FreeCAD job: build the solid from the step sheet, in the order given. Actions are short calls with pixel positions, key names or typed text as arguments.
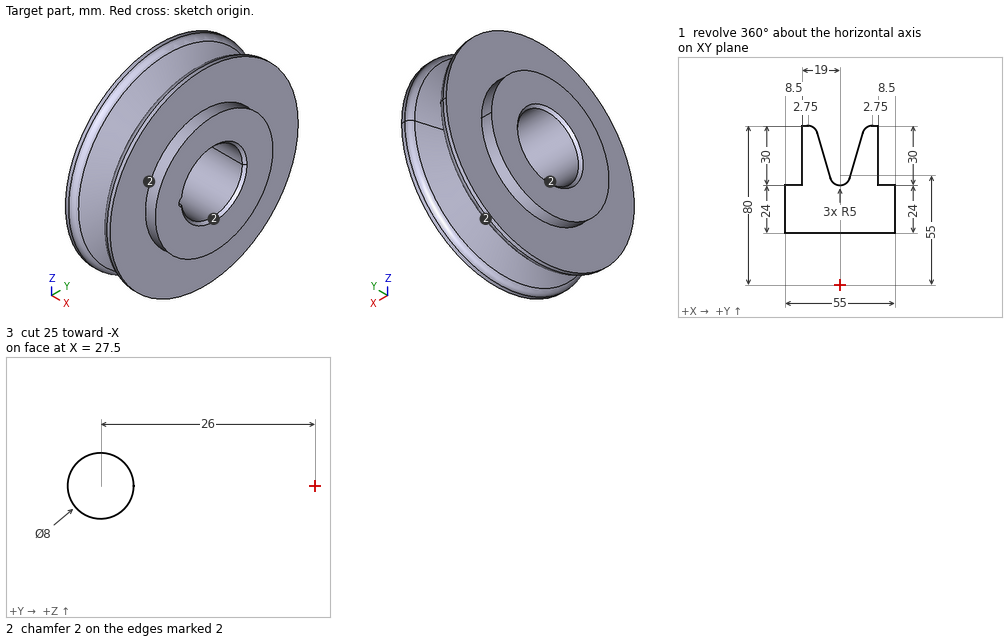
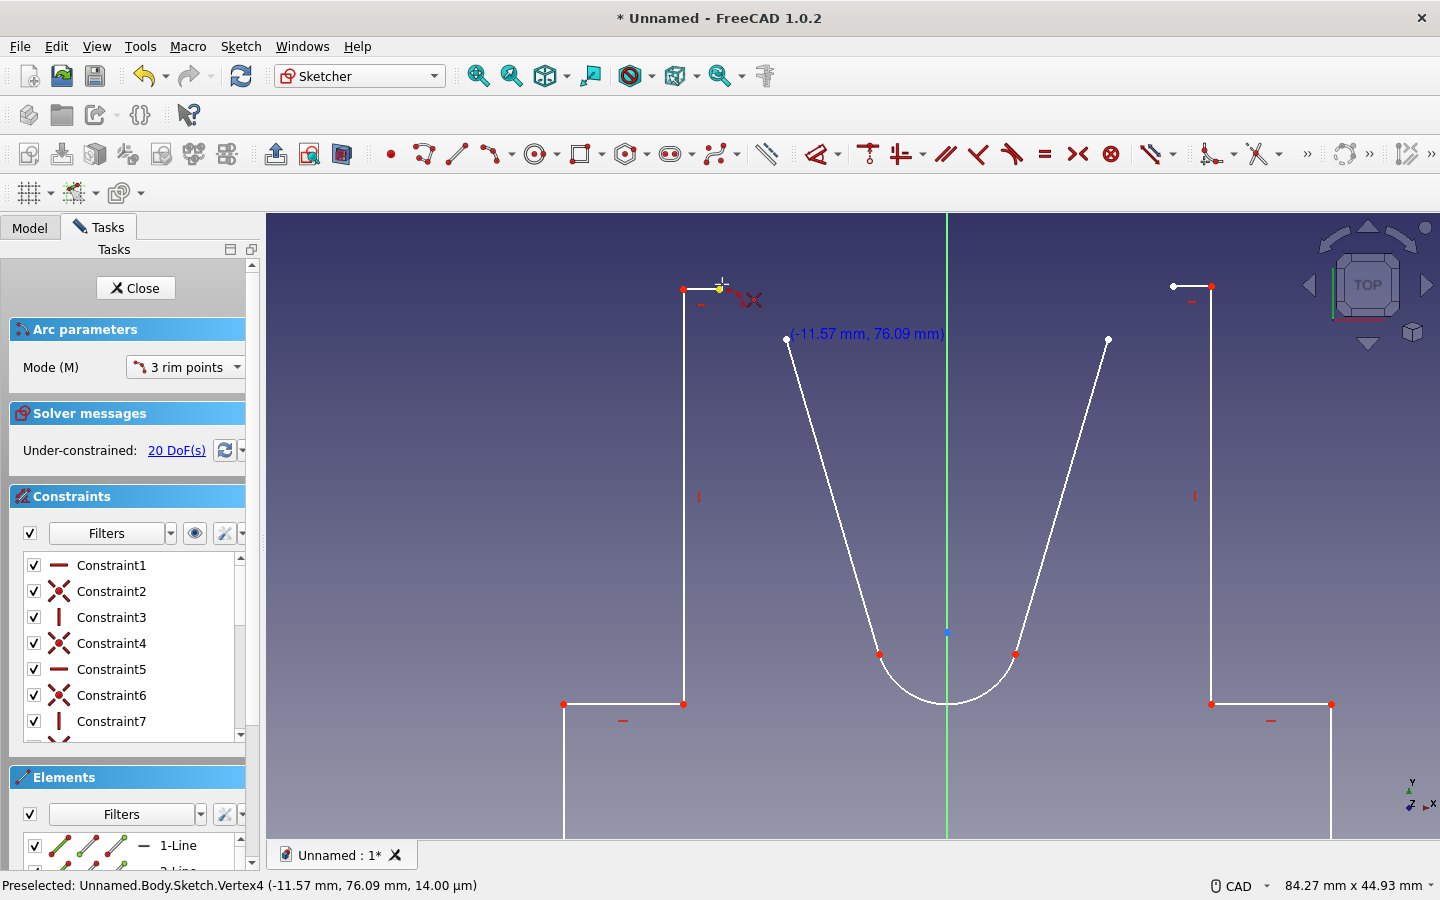
click(720, 289)
click(763, 298)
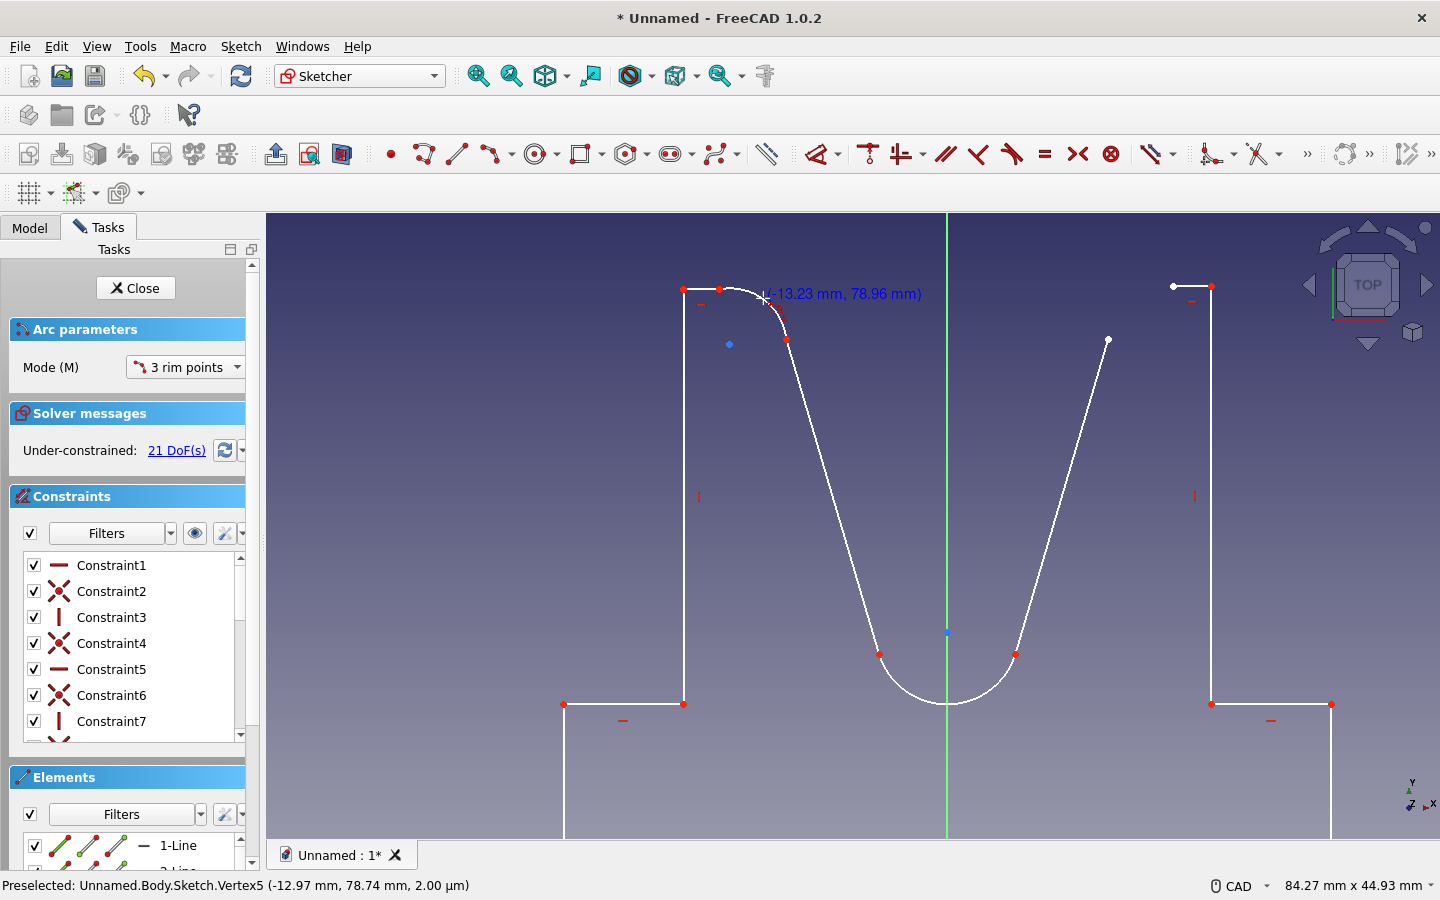
click(1173, 286)
click(1108, 339)
click(1132, 298)
key(Escape)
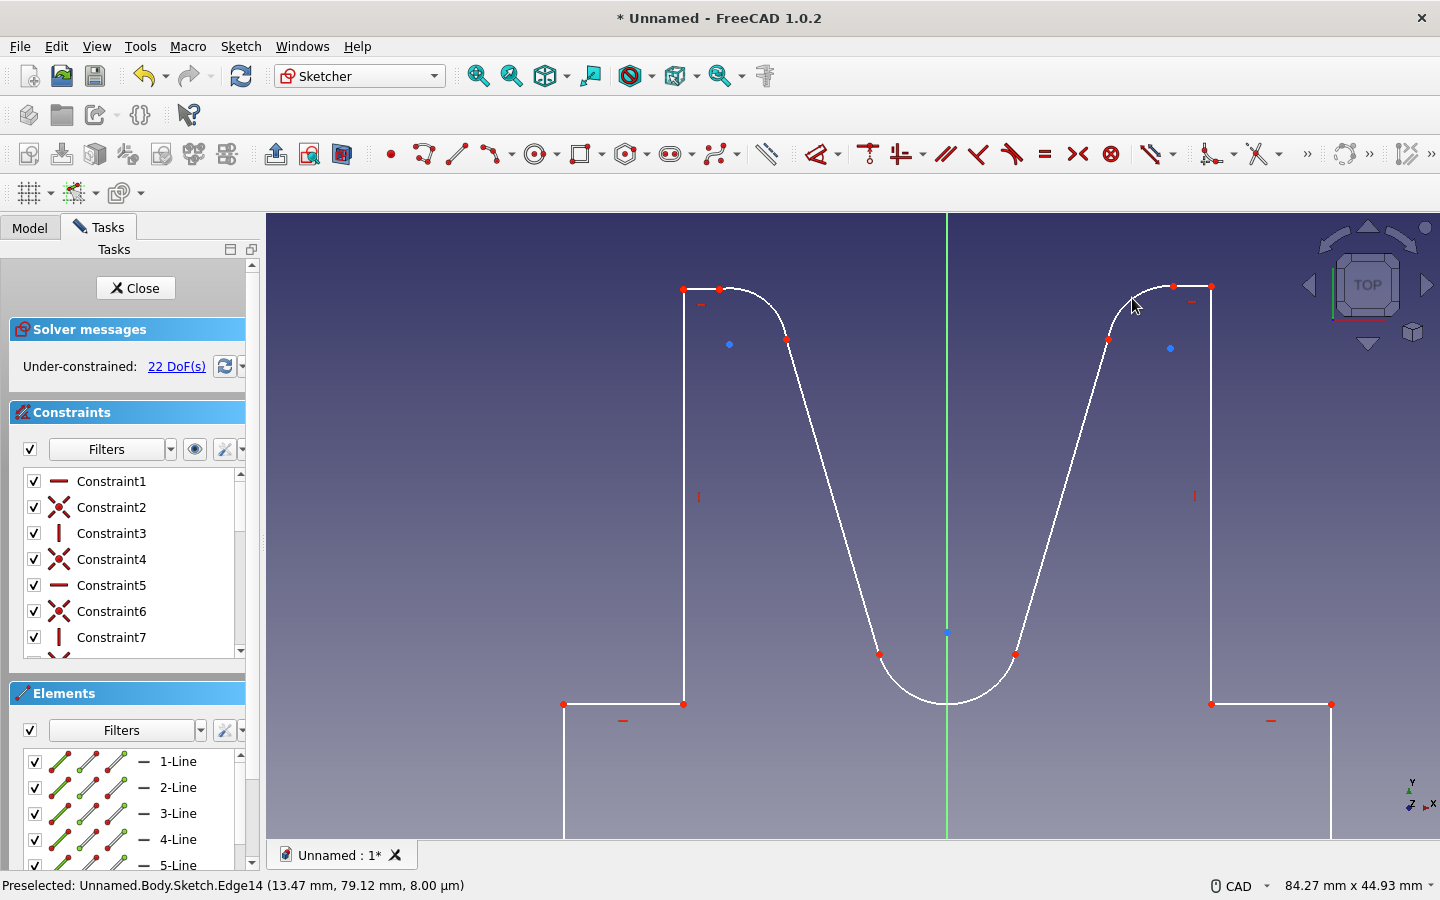
click(1080, 434)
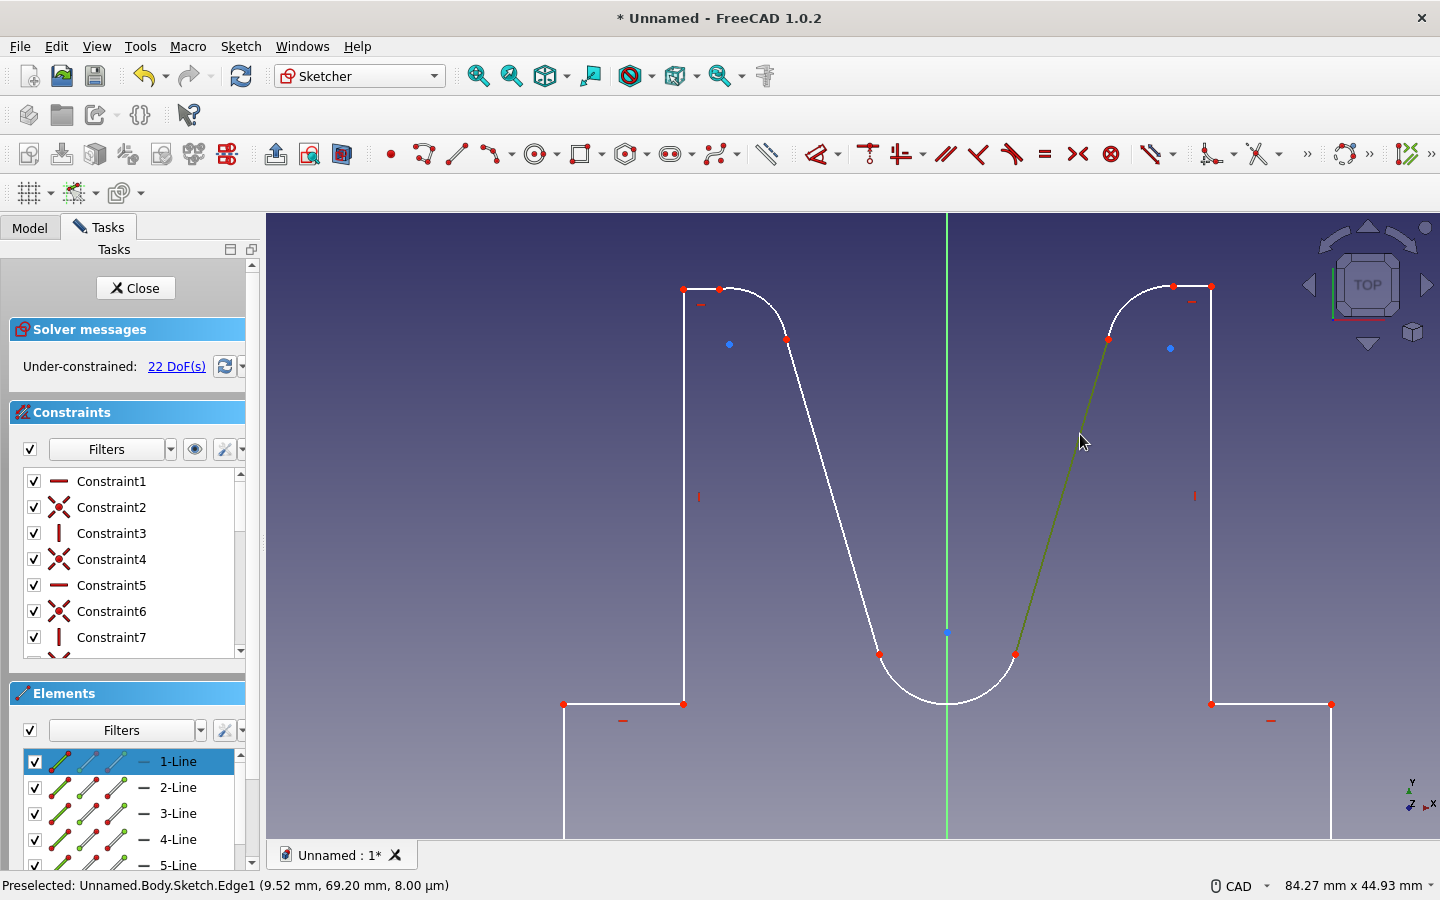
click(913, 695)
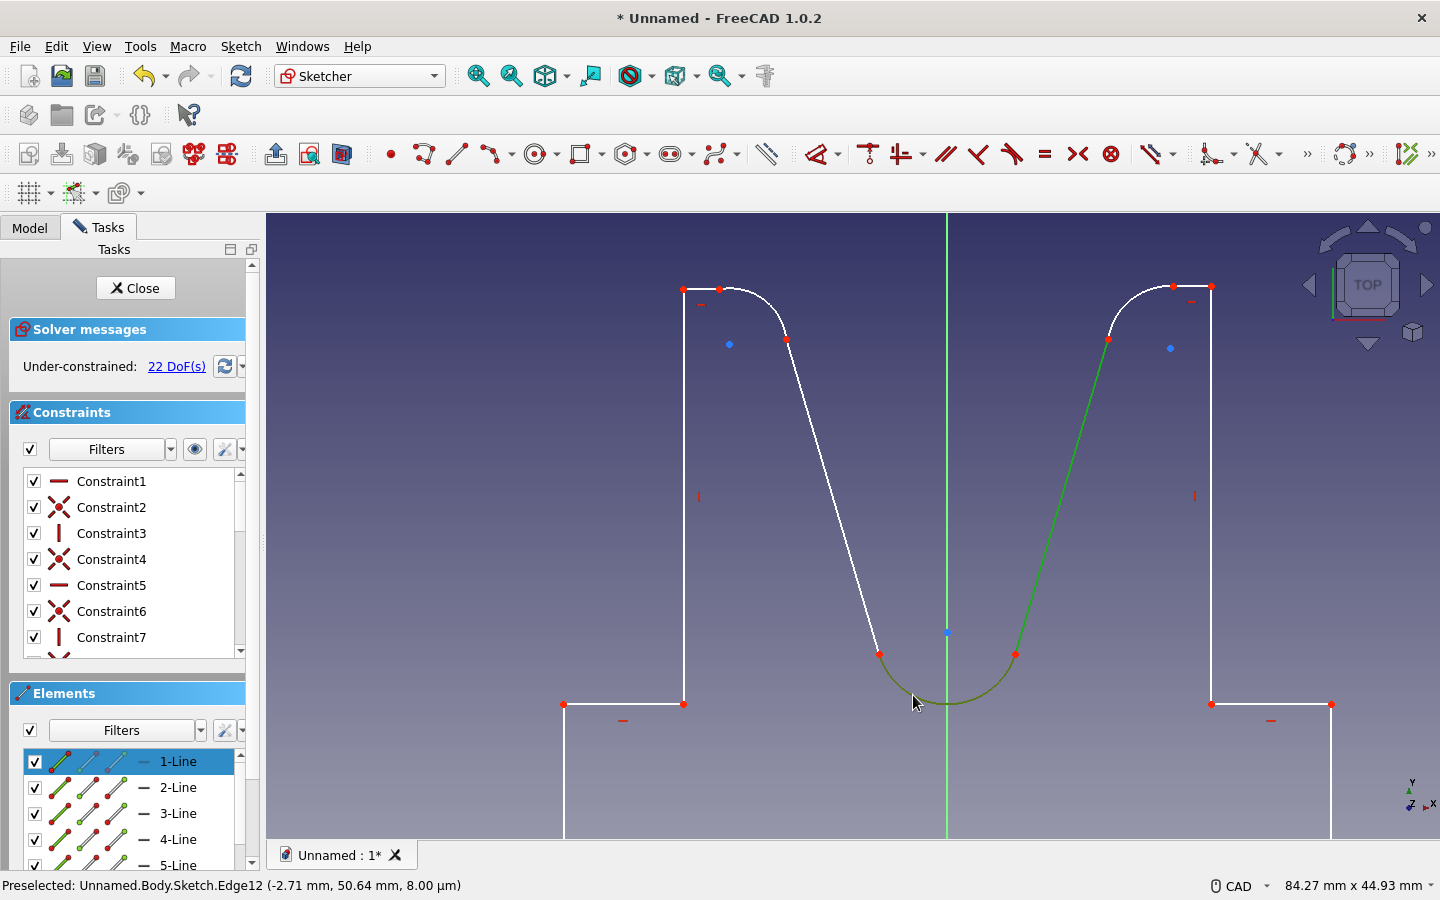
key(t)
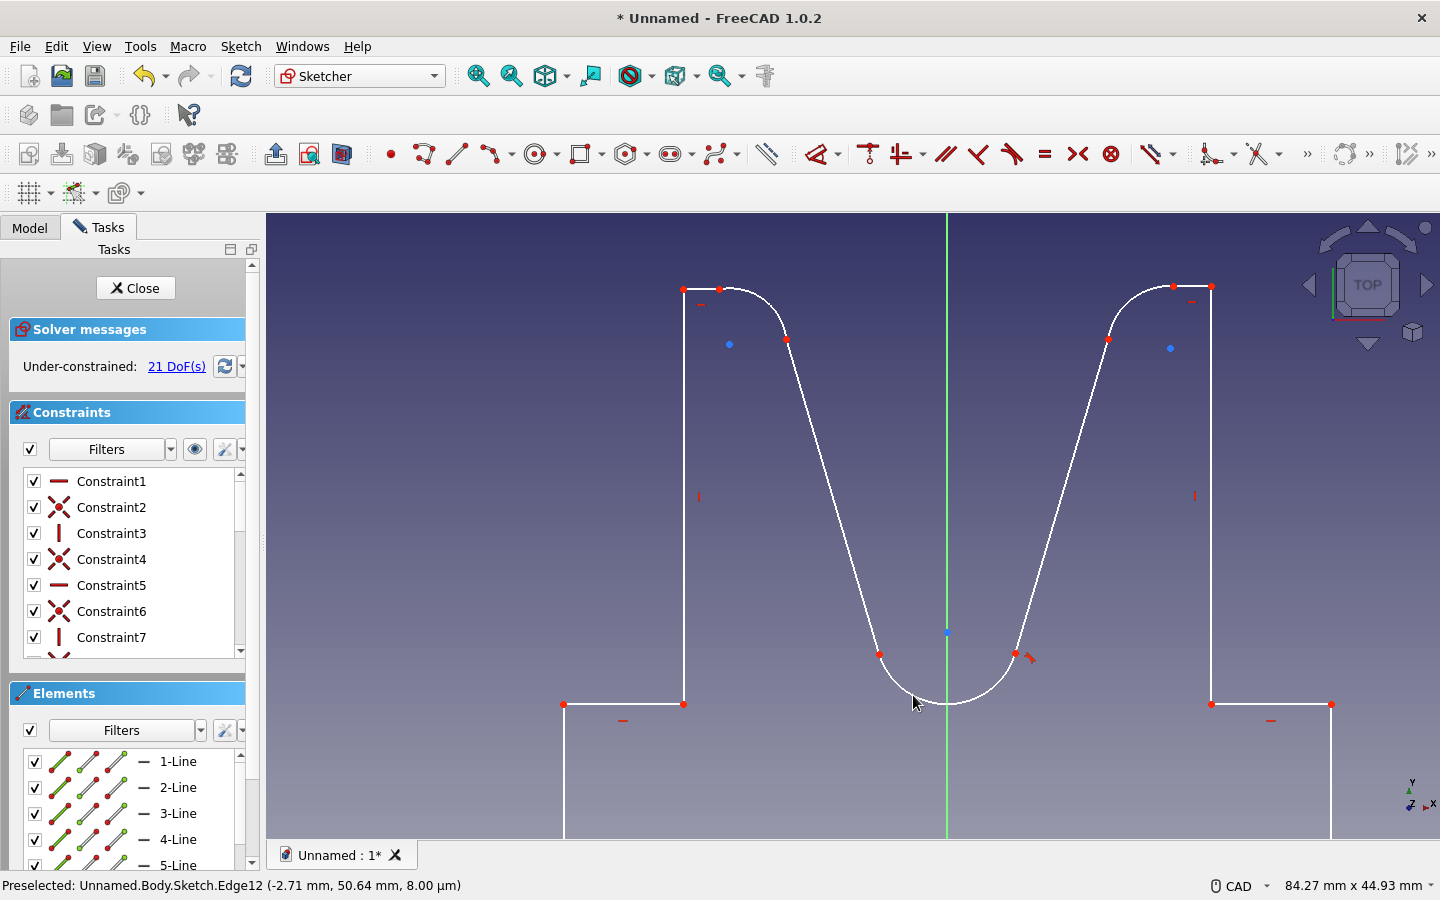
click(1080, 433)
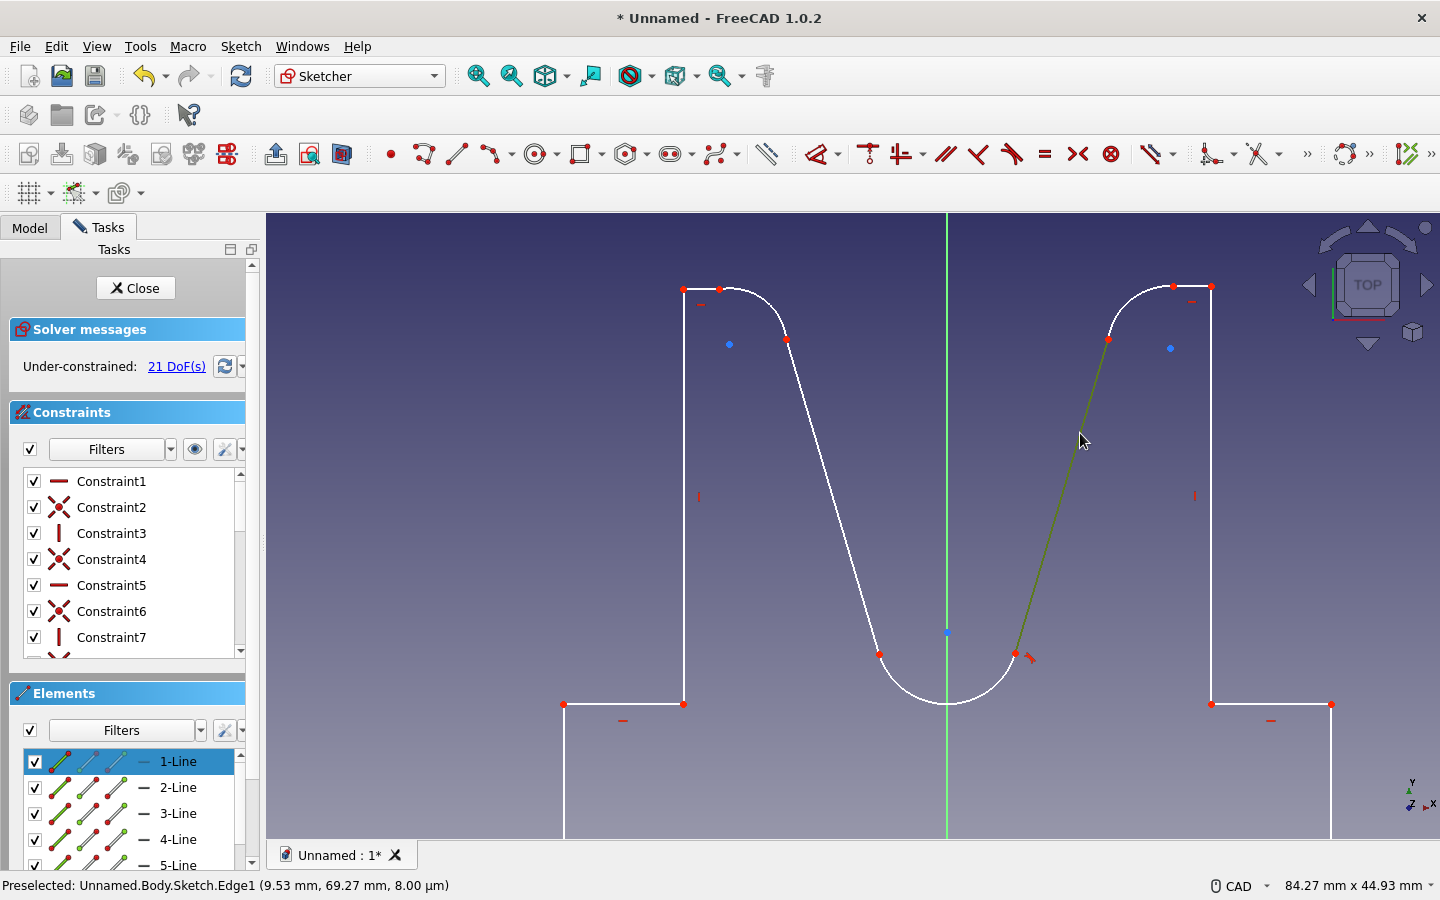
click(1146, 291)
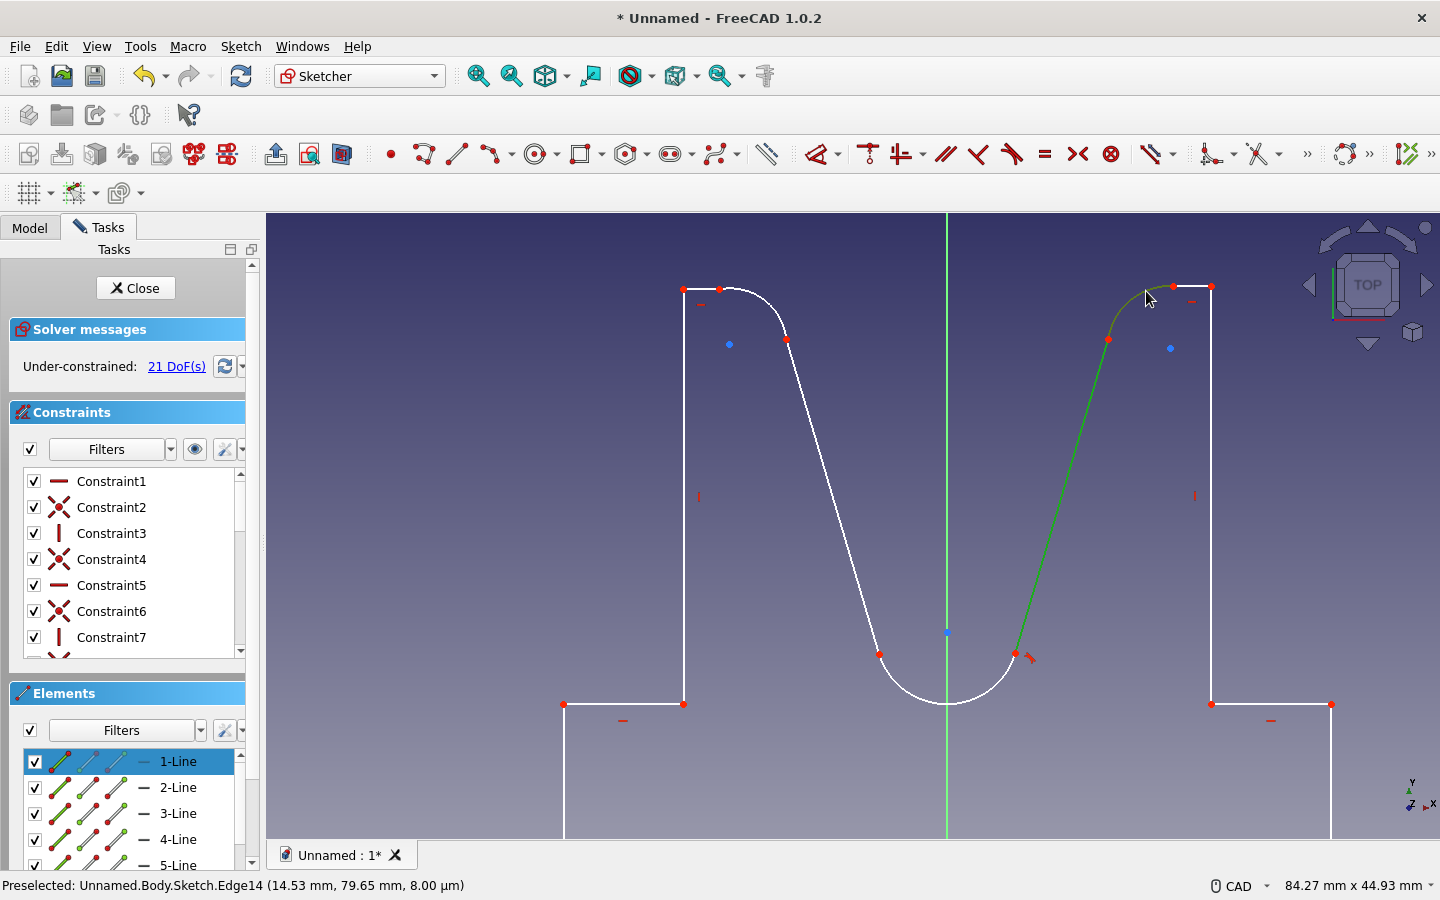
key(t)